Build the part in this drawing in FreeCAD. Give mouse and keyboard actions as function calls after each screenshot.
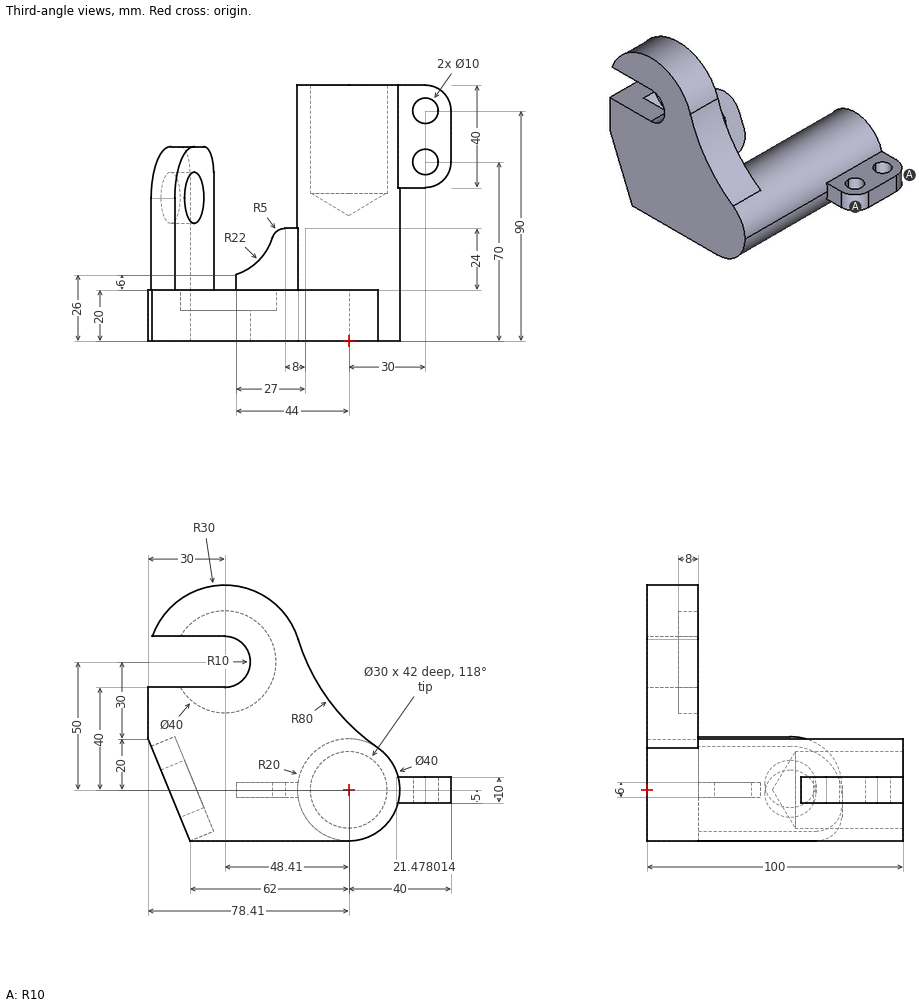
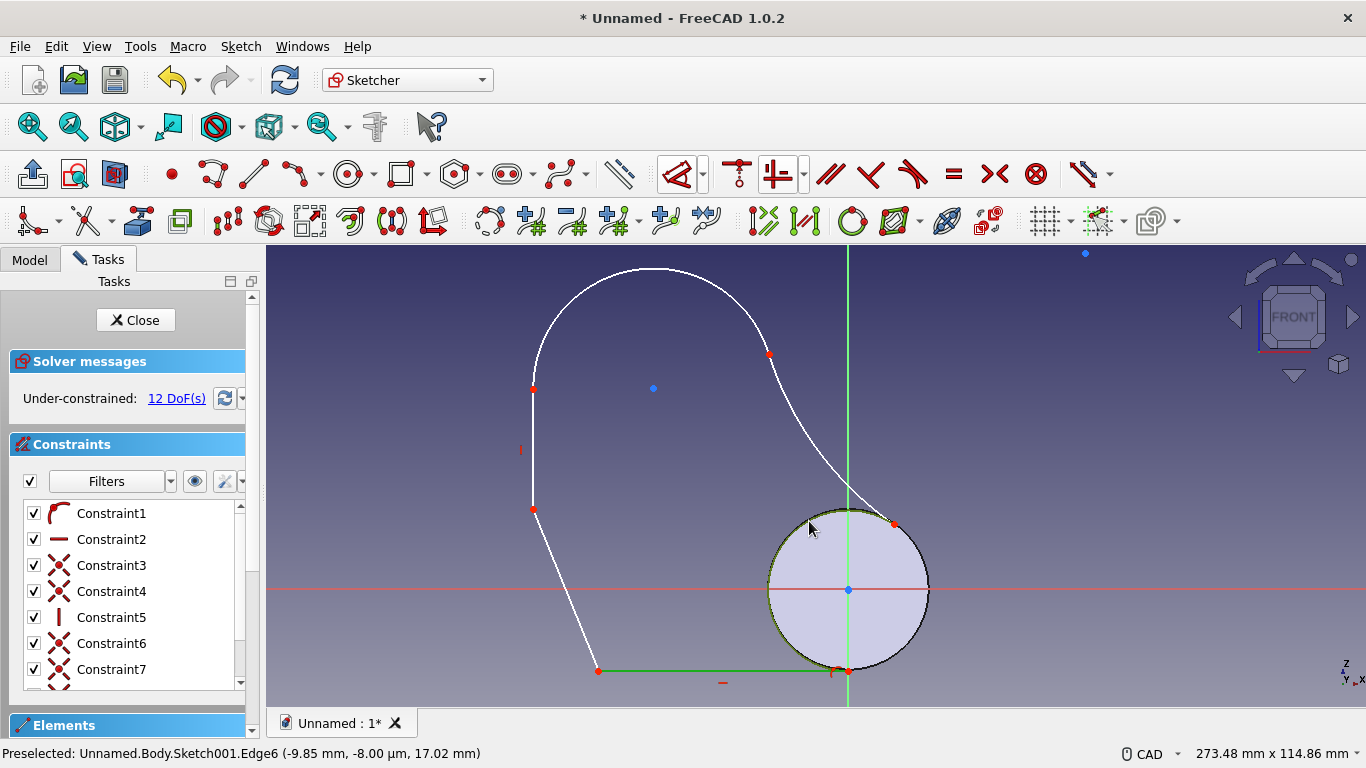
key(t)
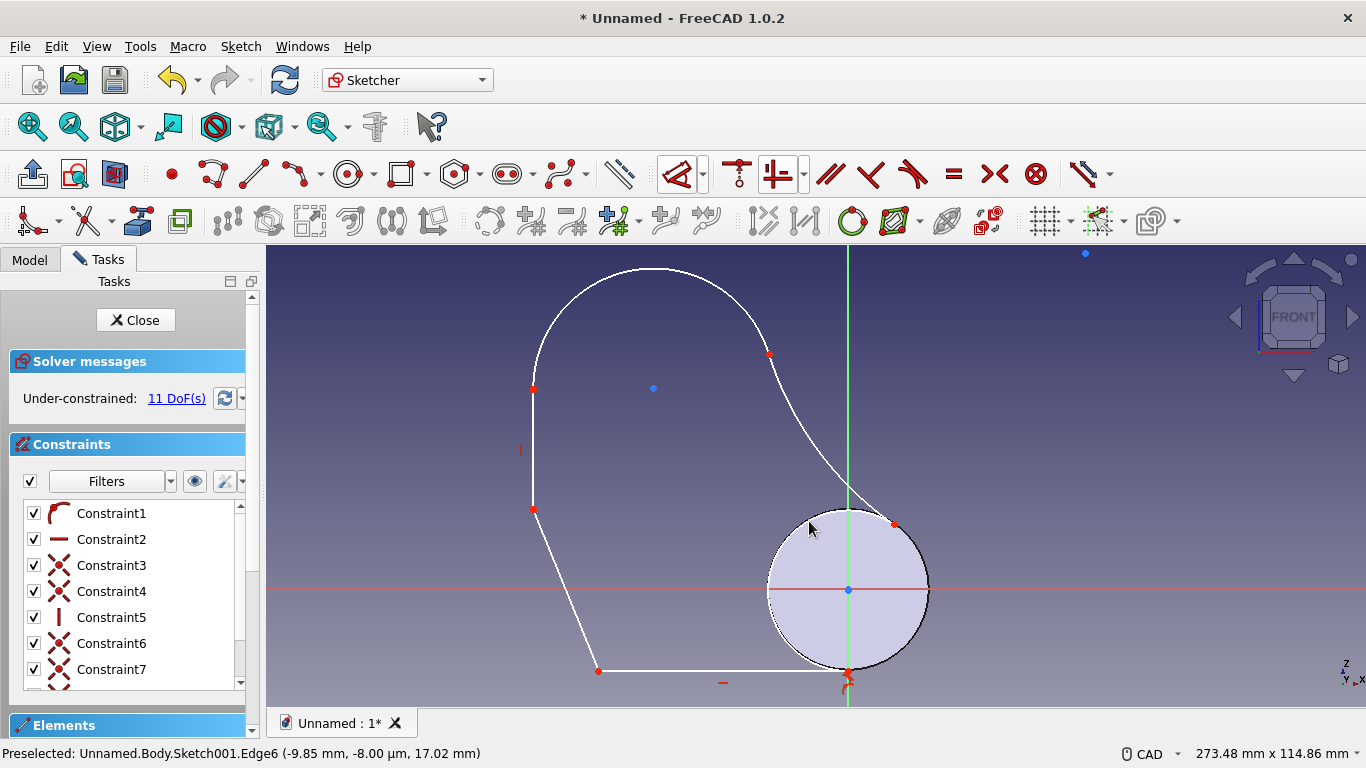
click(533, 474)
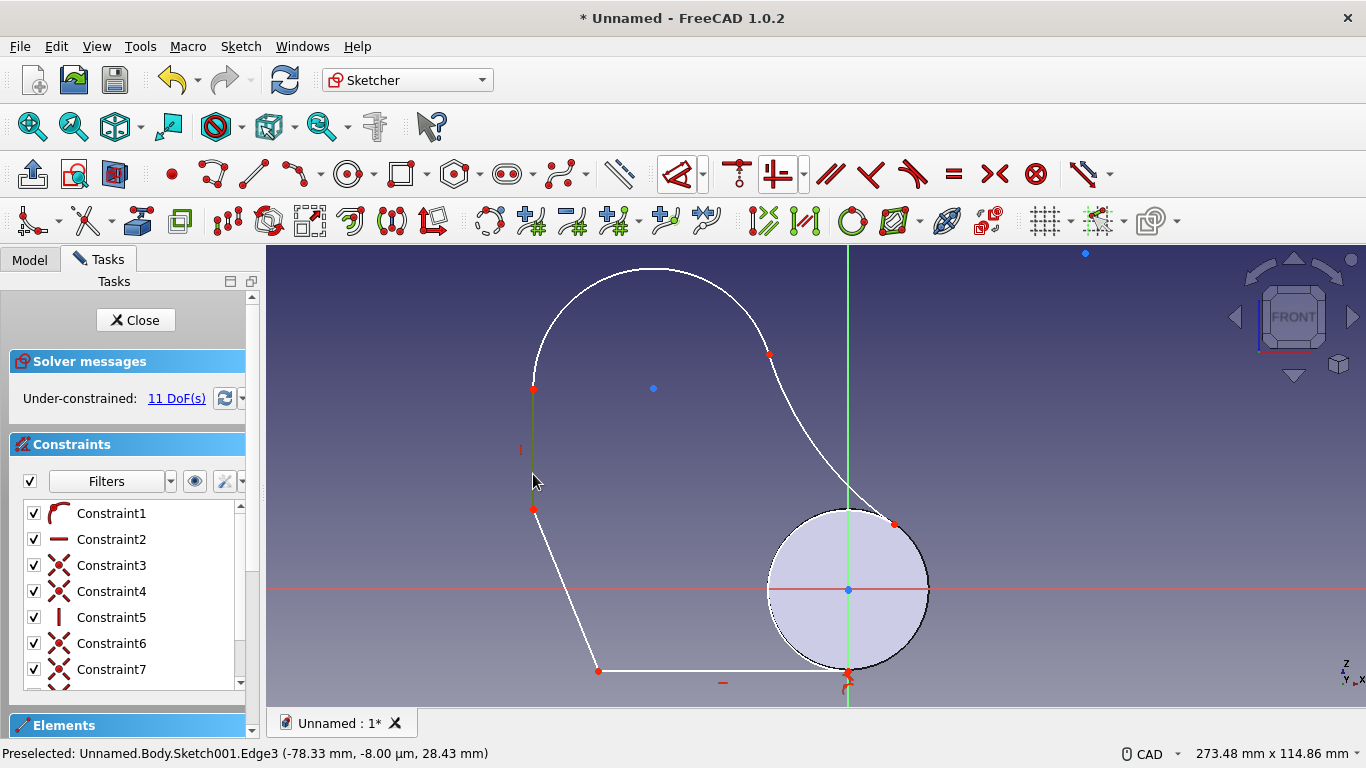
click(703, 279)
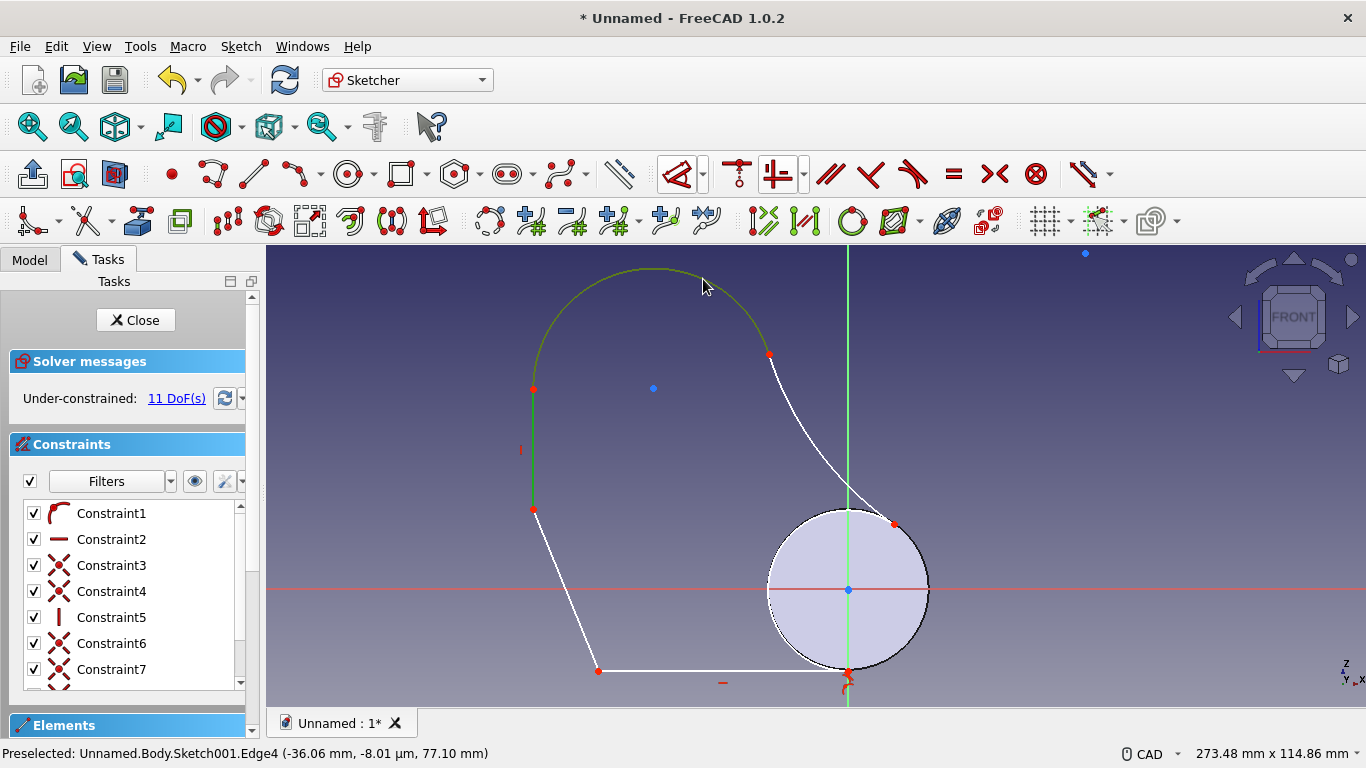
key(t)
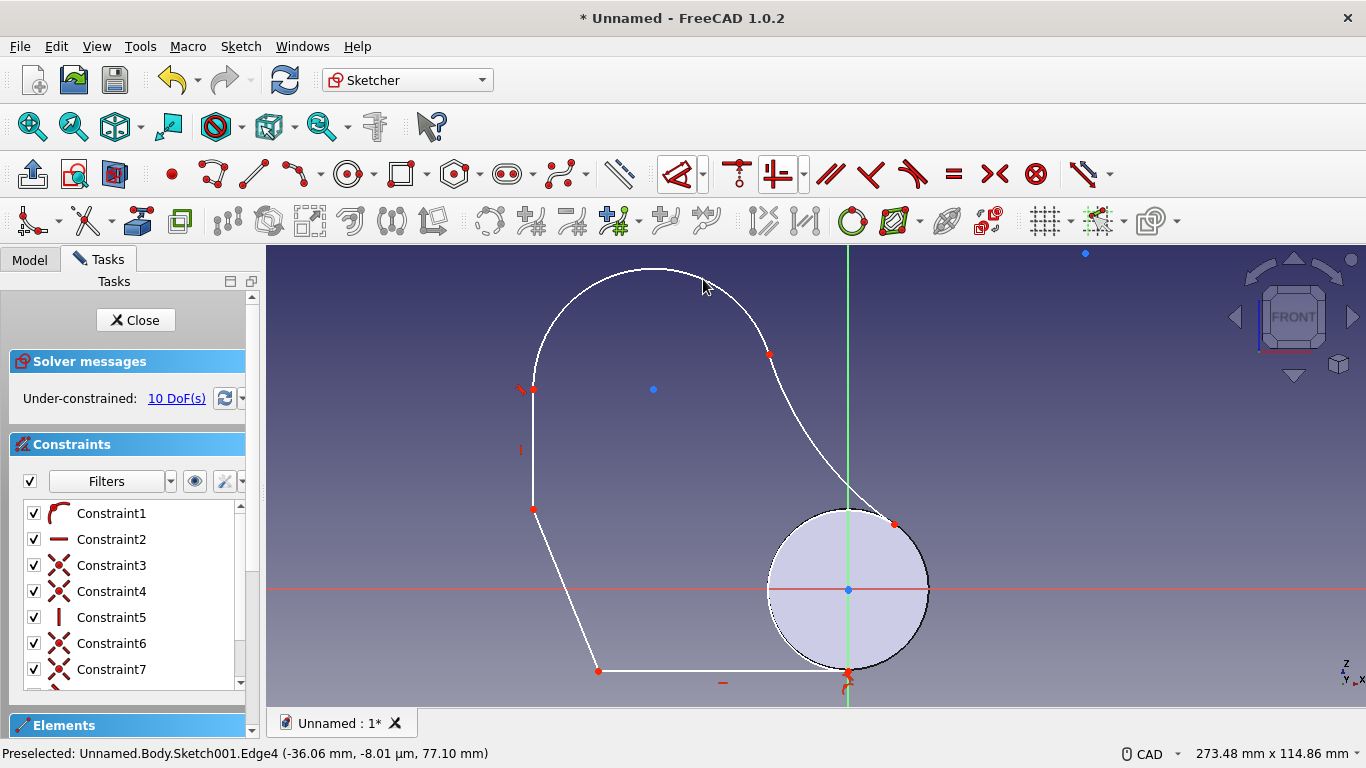
click(703, 280)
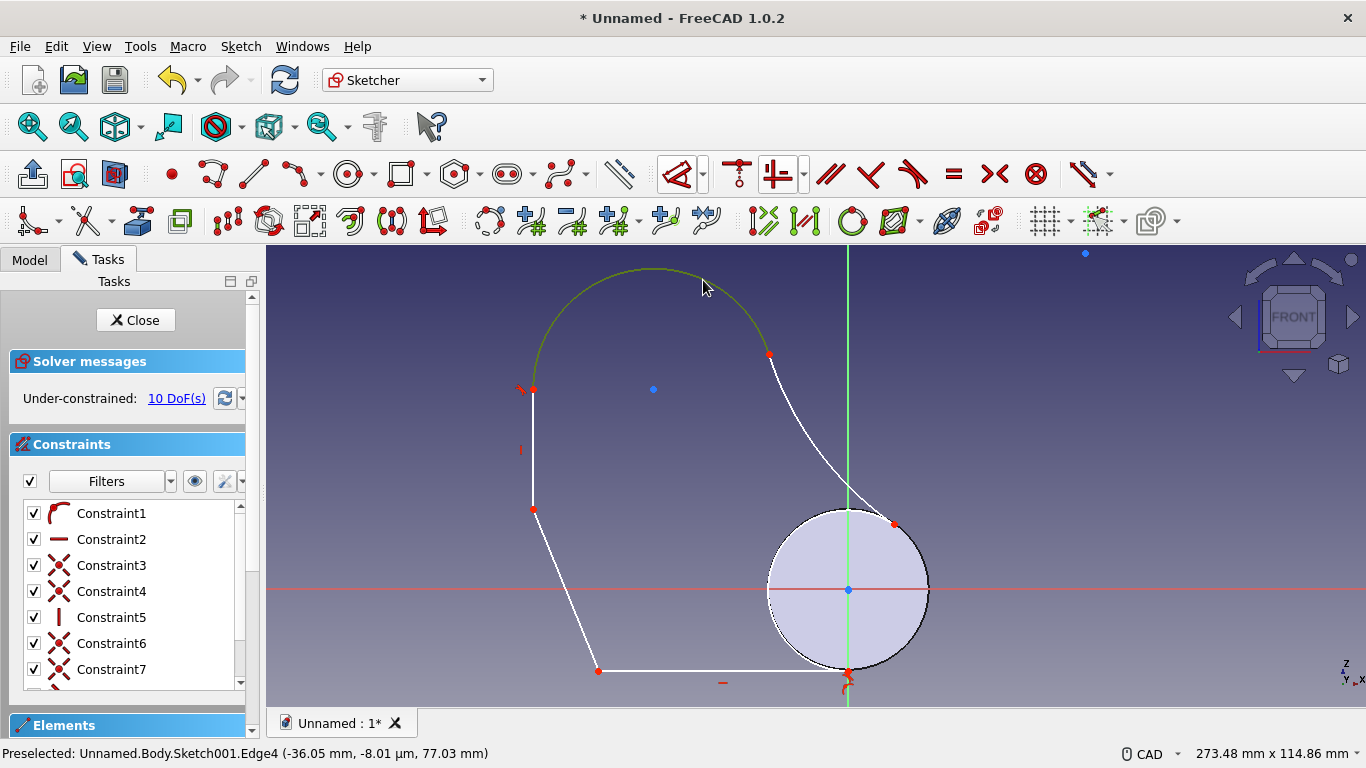
click(795, 414)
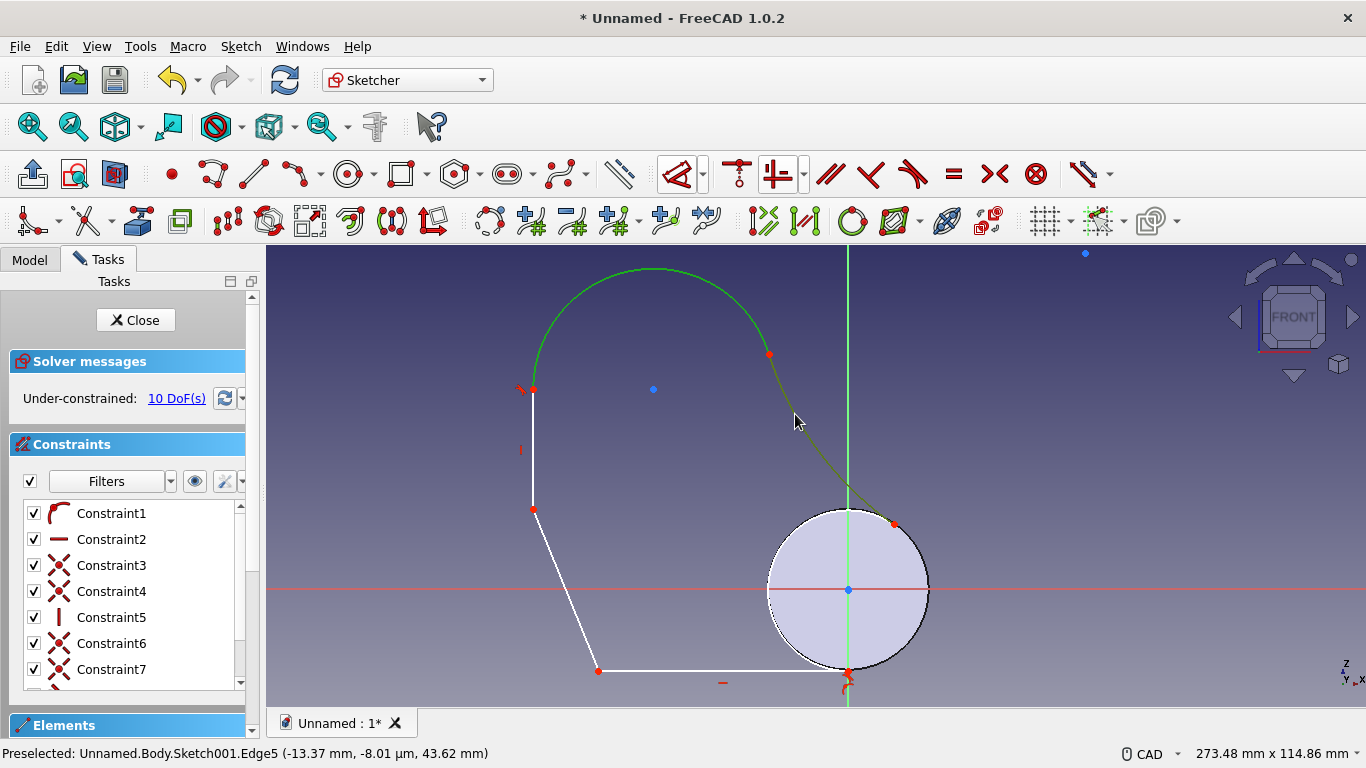
key(t)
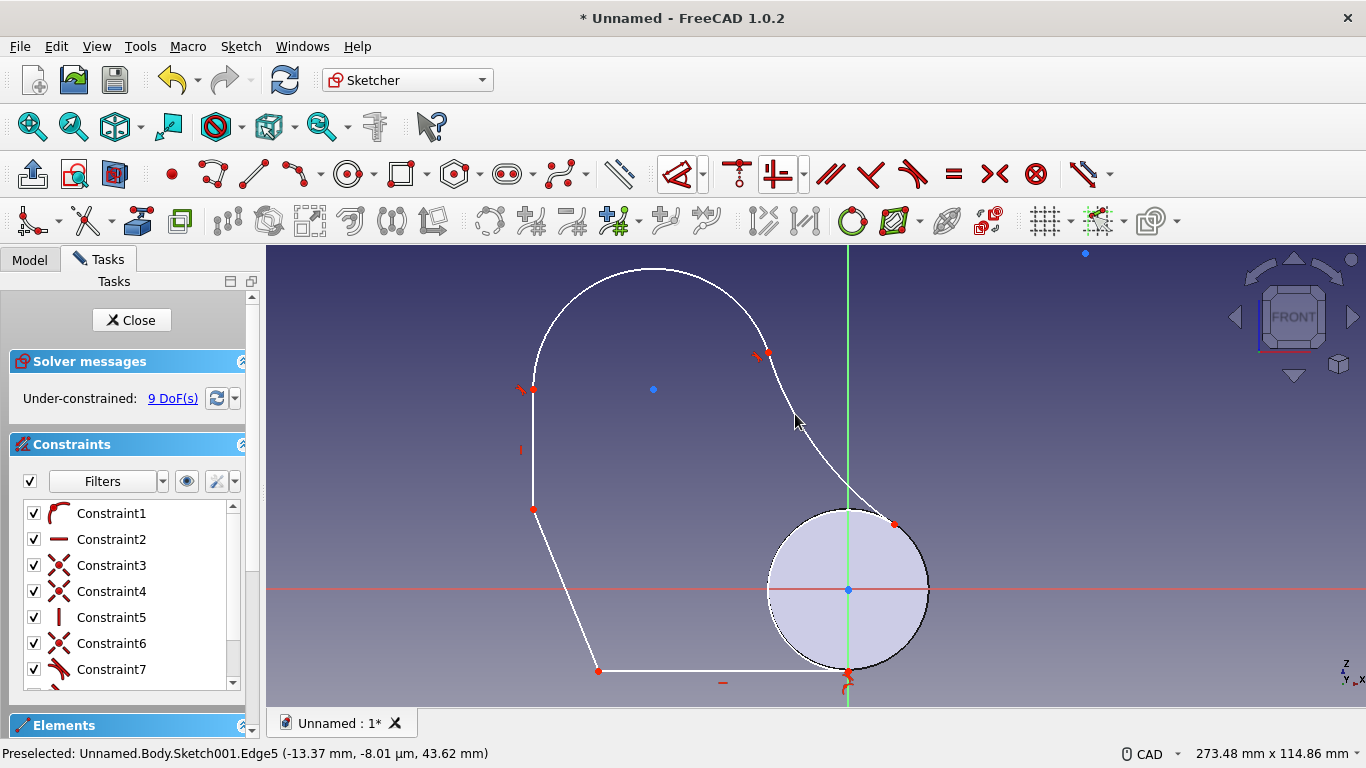
click(794, 413)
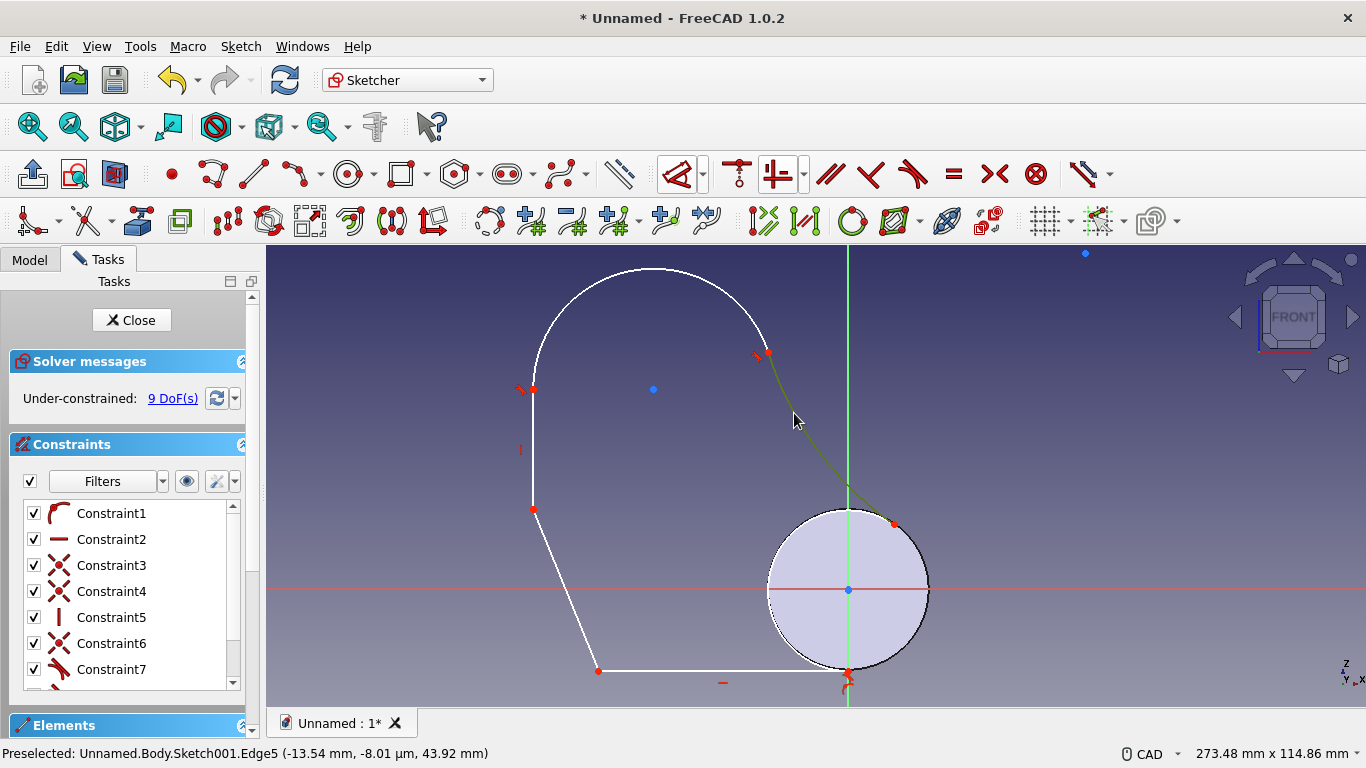
click(809, 521)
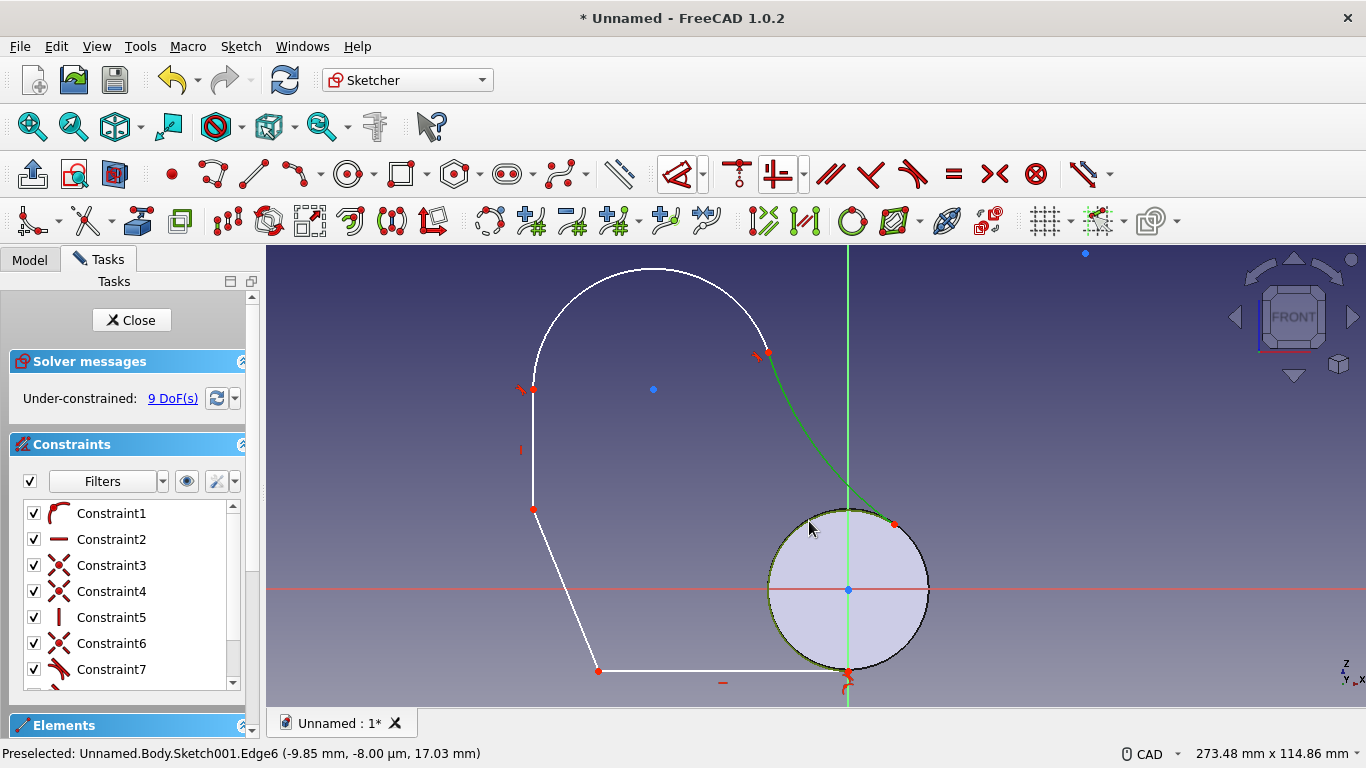
key(t)